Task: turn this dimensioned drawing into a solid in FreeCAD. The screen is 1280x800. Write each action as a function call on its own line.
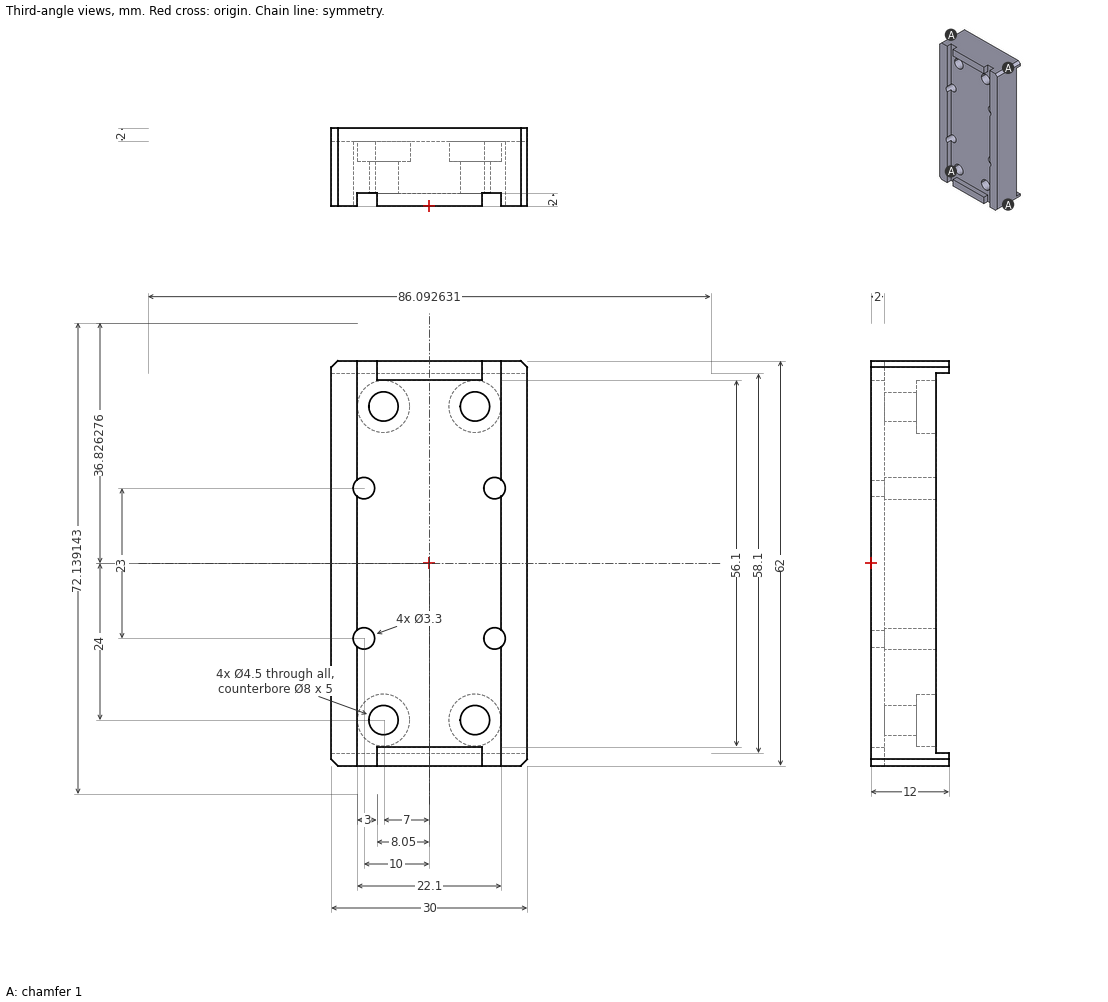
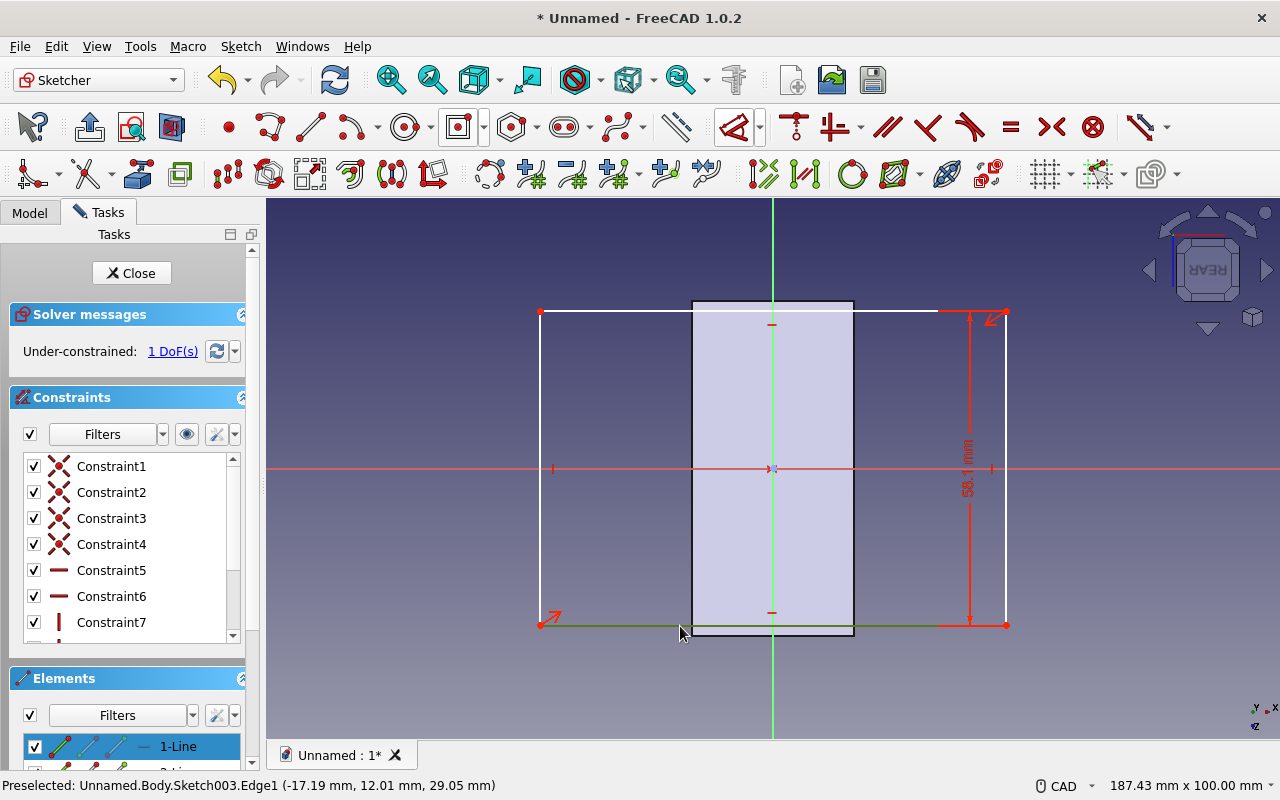
click(760, 128)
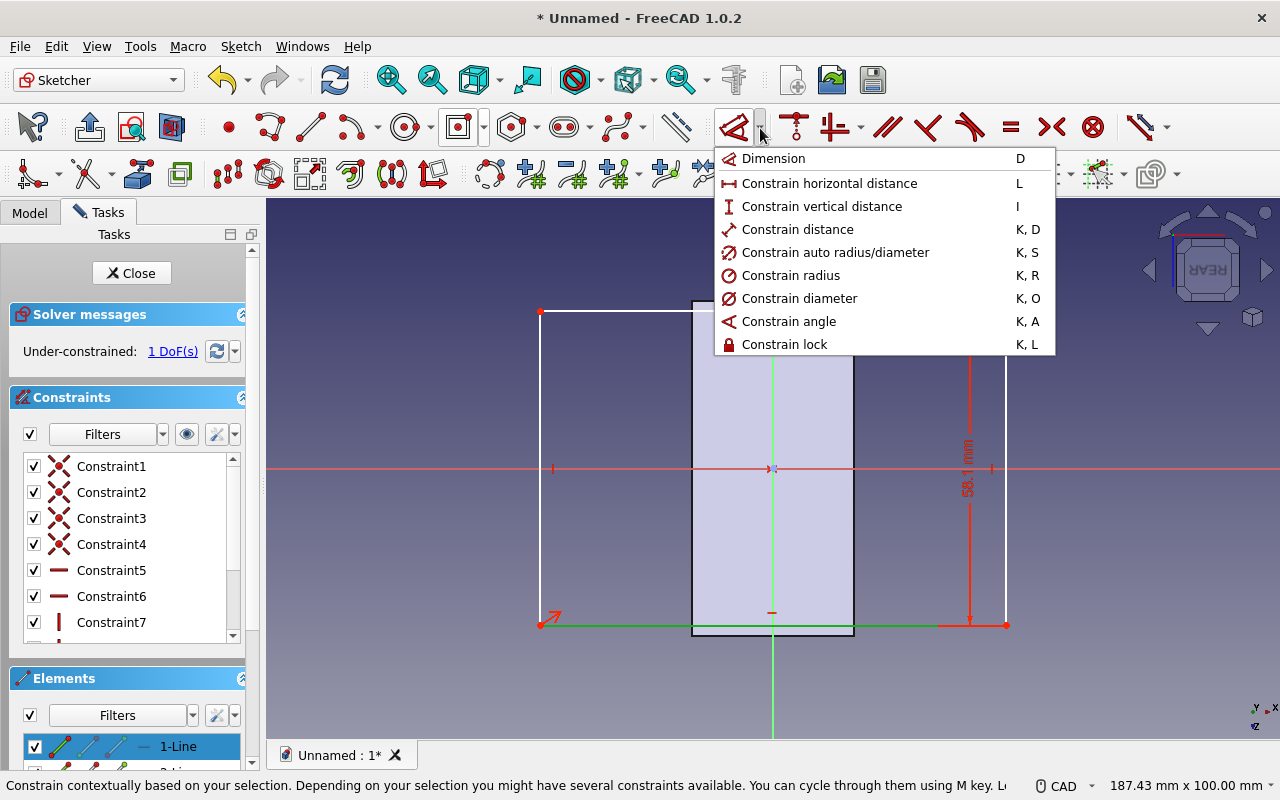
click(885, 184)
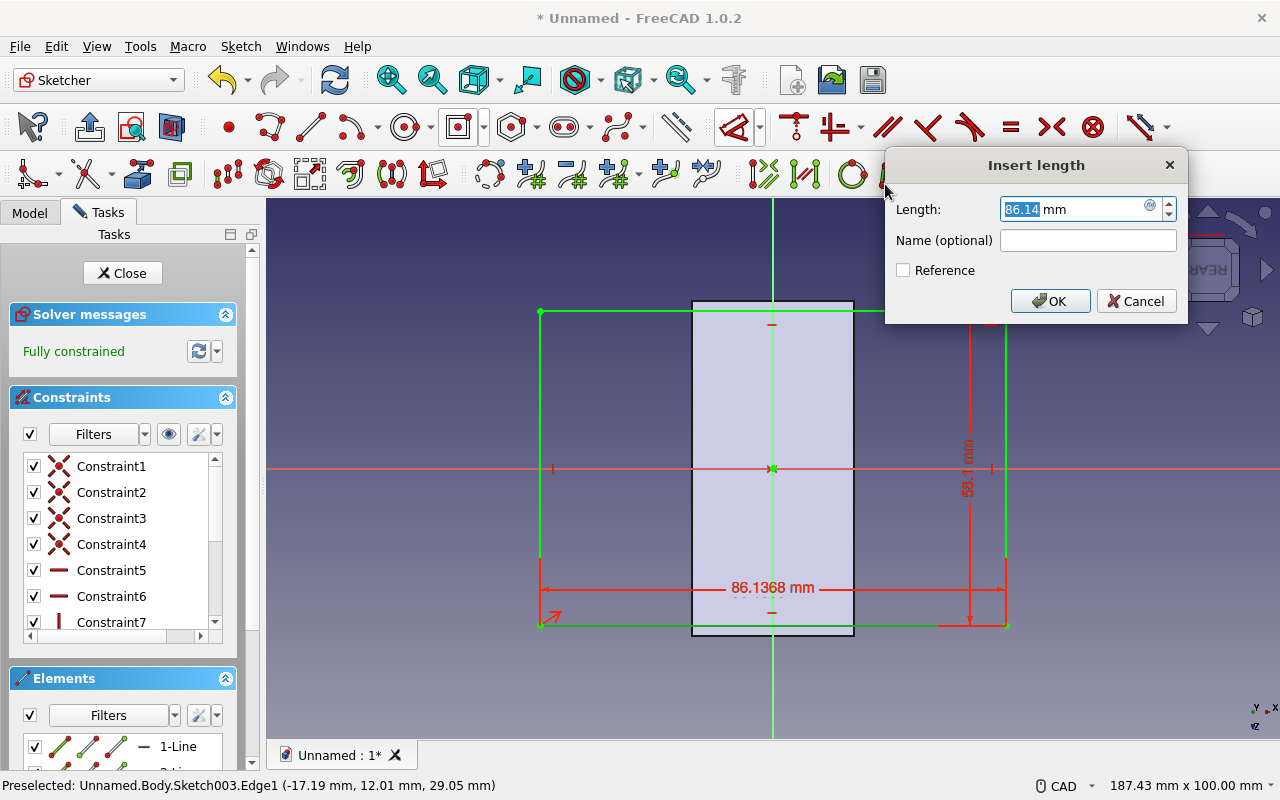
text(86.092631)
key(Return)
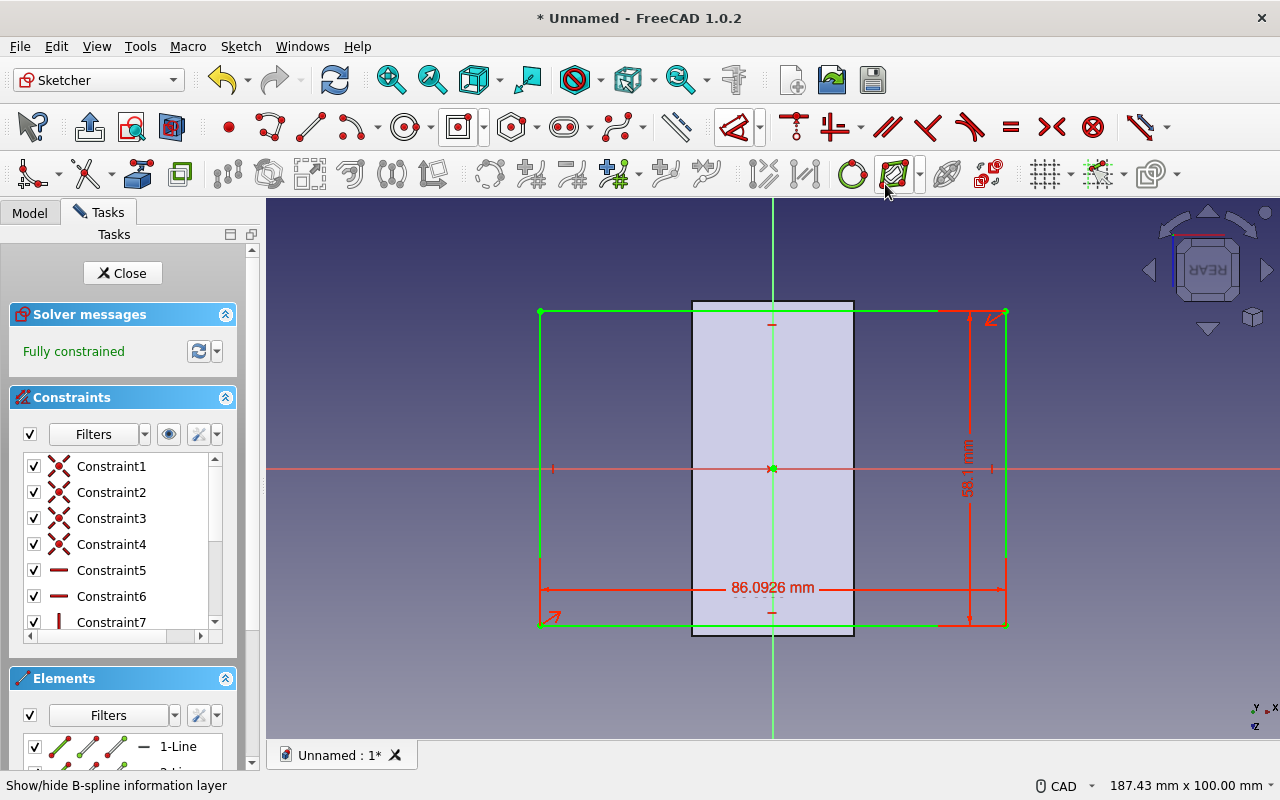
click(123, 273)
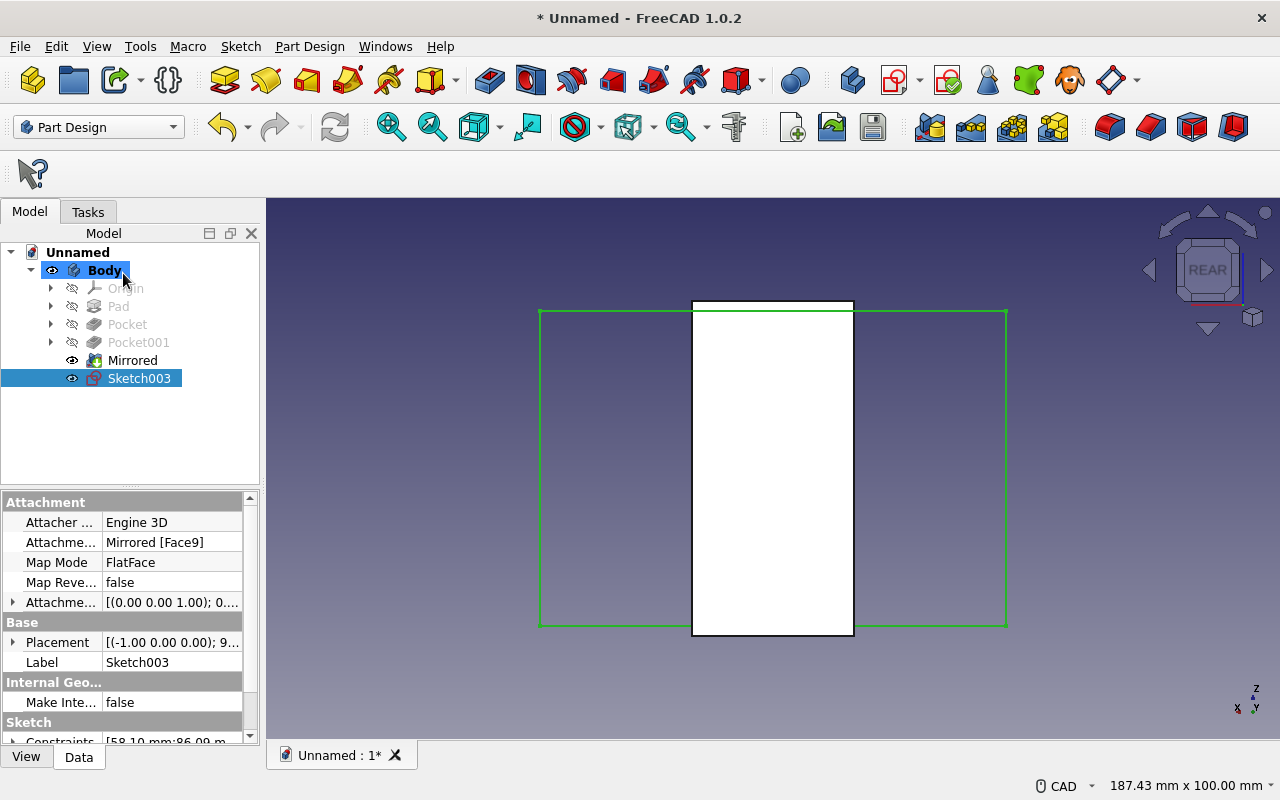
click(490, 80)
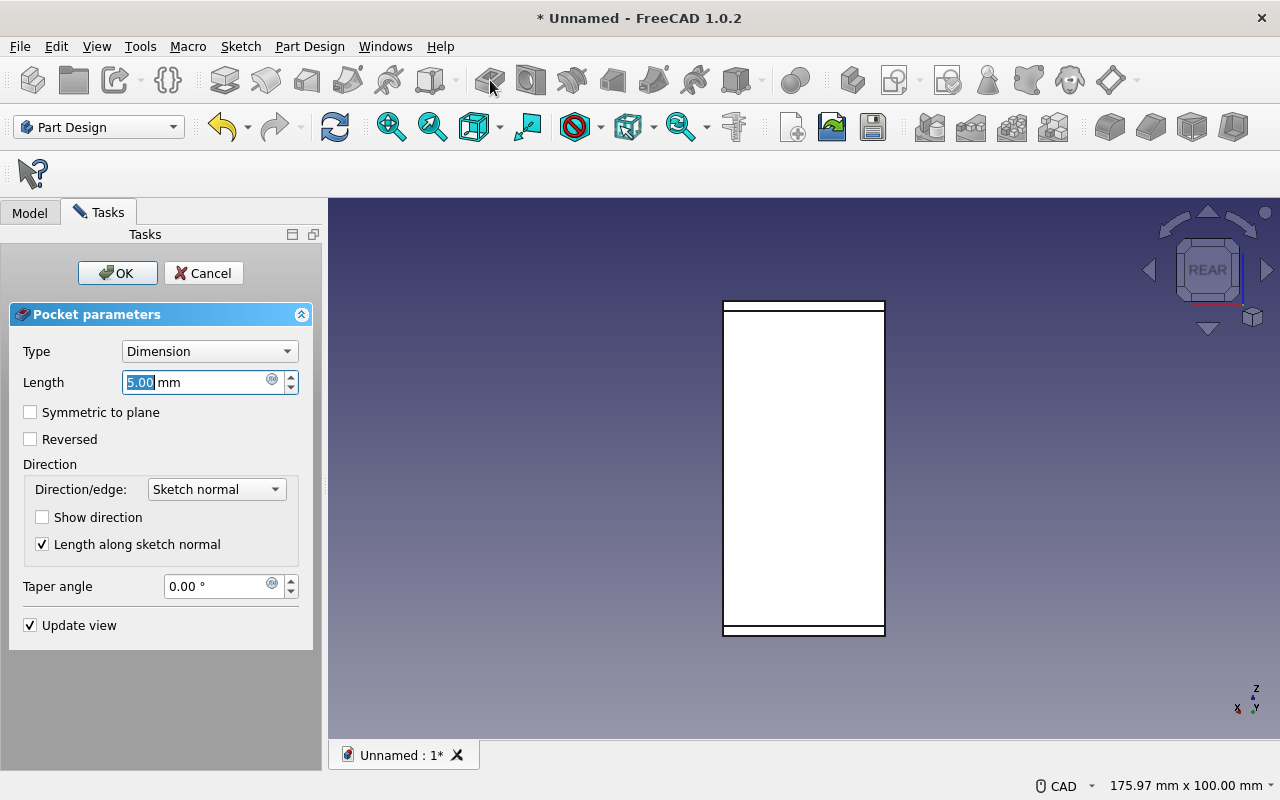
text(2)
key(Tab)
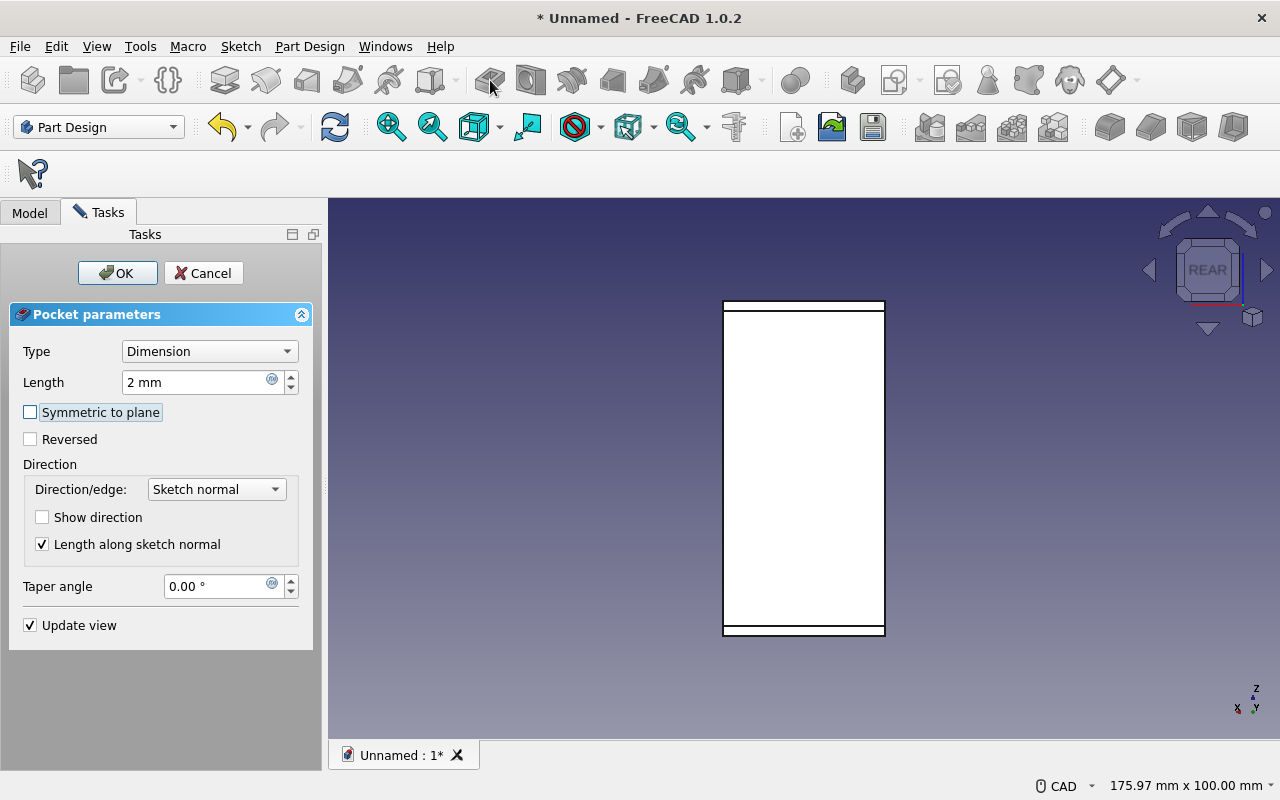
click(118, 273)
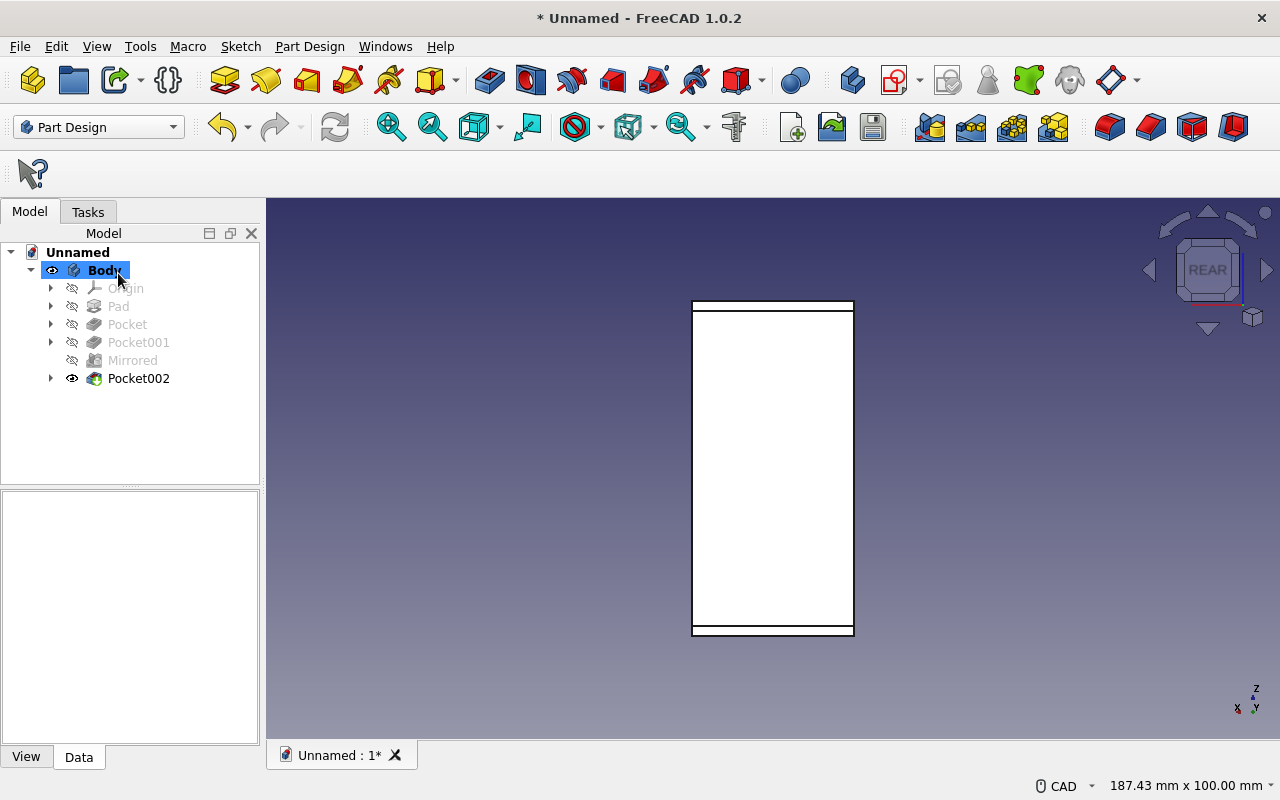
click(773, 512)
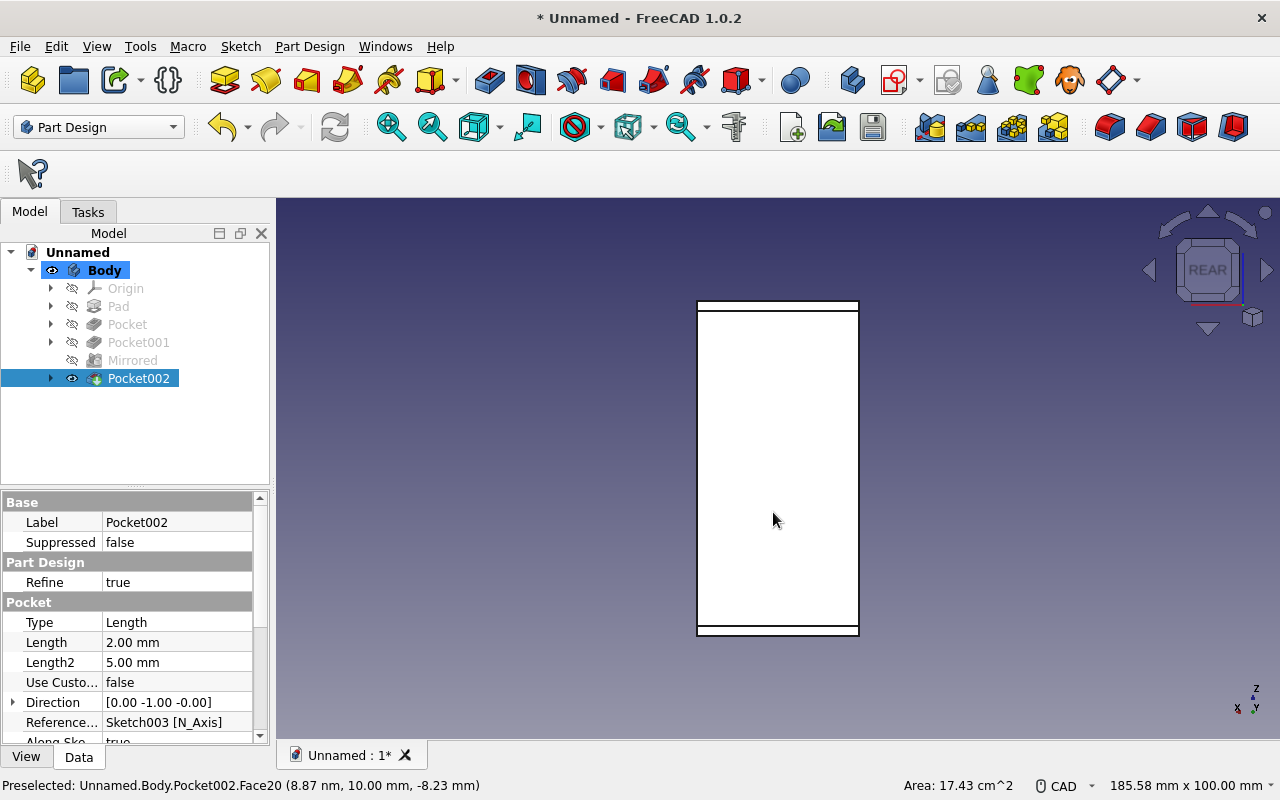
click(894, 80)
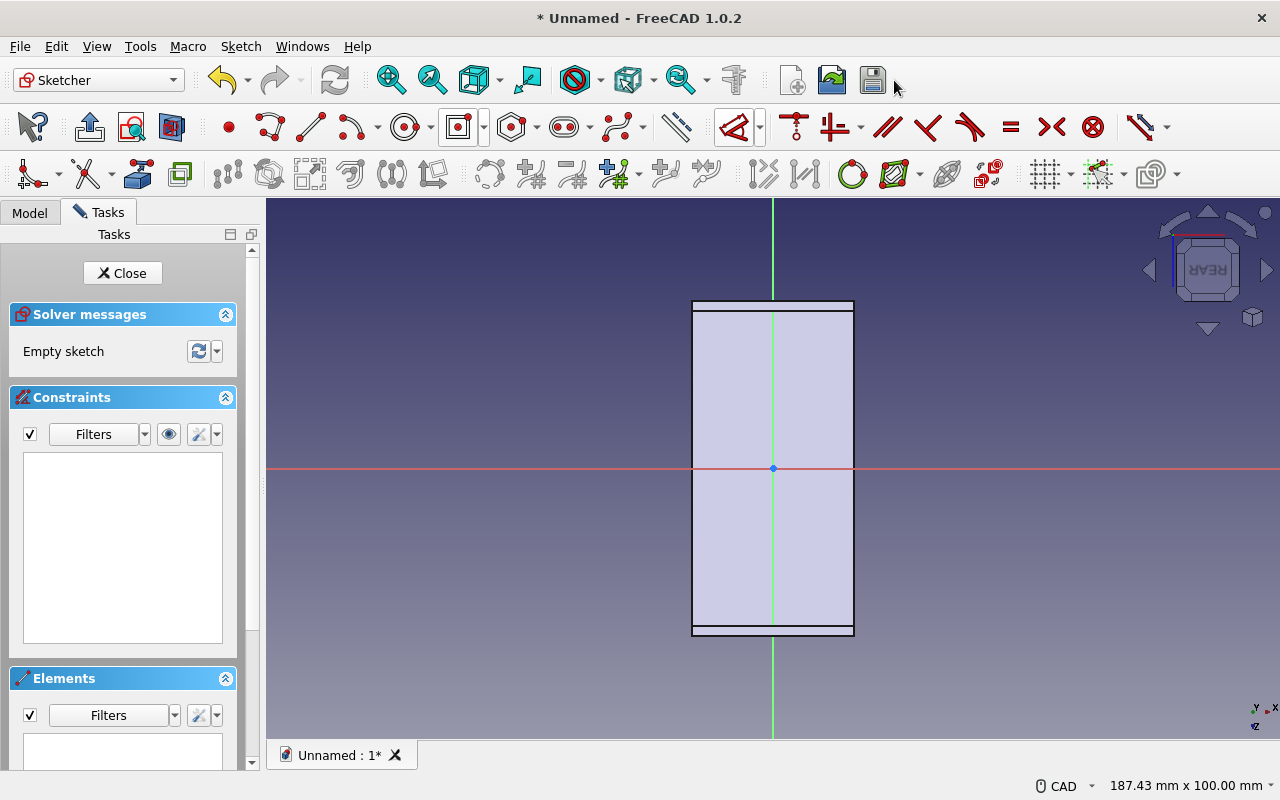
click(172, 128)